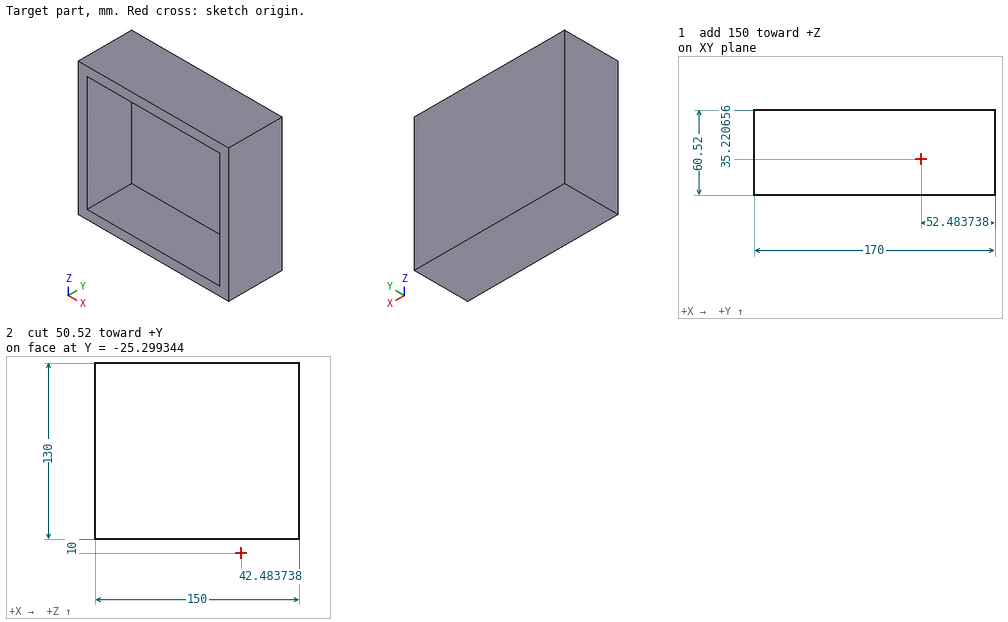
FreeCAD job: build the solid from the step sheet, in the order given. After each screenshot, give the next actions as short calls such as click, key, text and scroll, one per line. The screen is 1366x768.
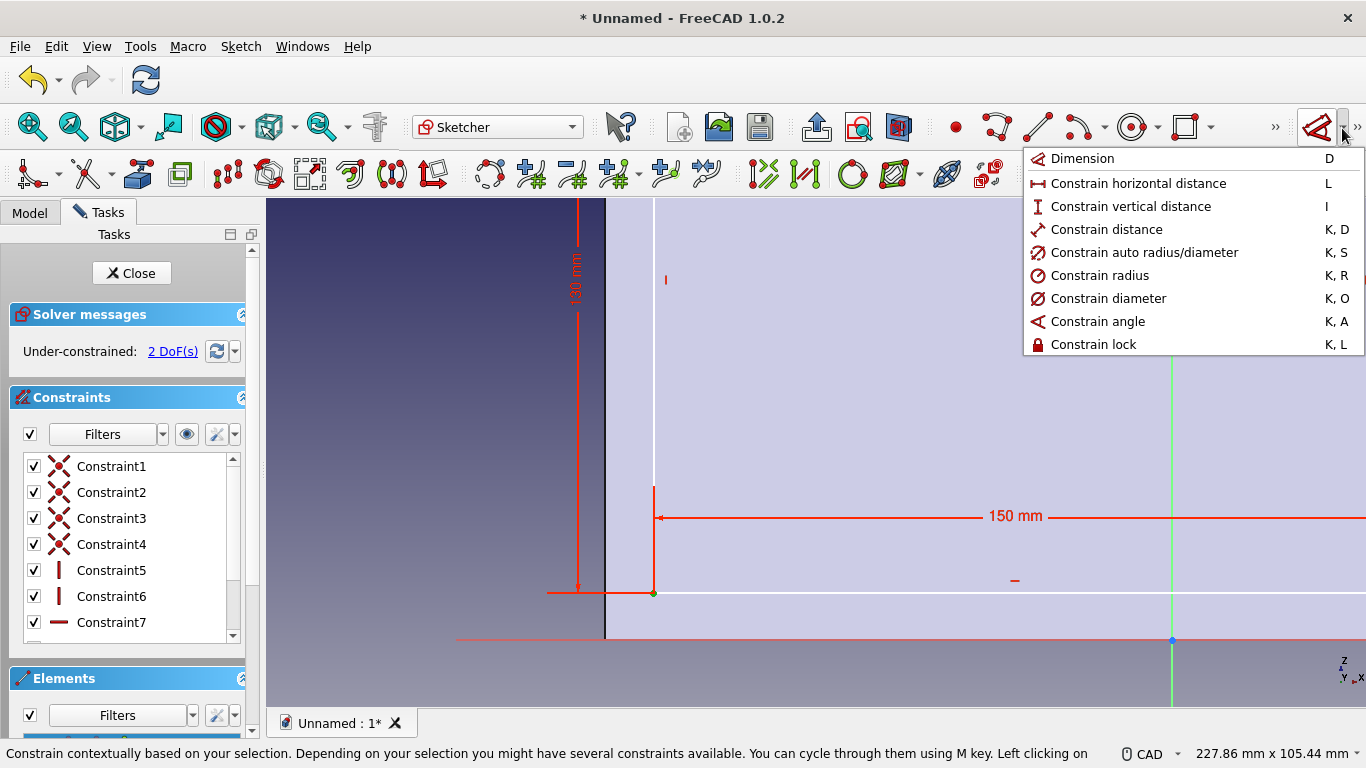
click(1194, 206)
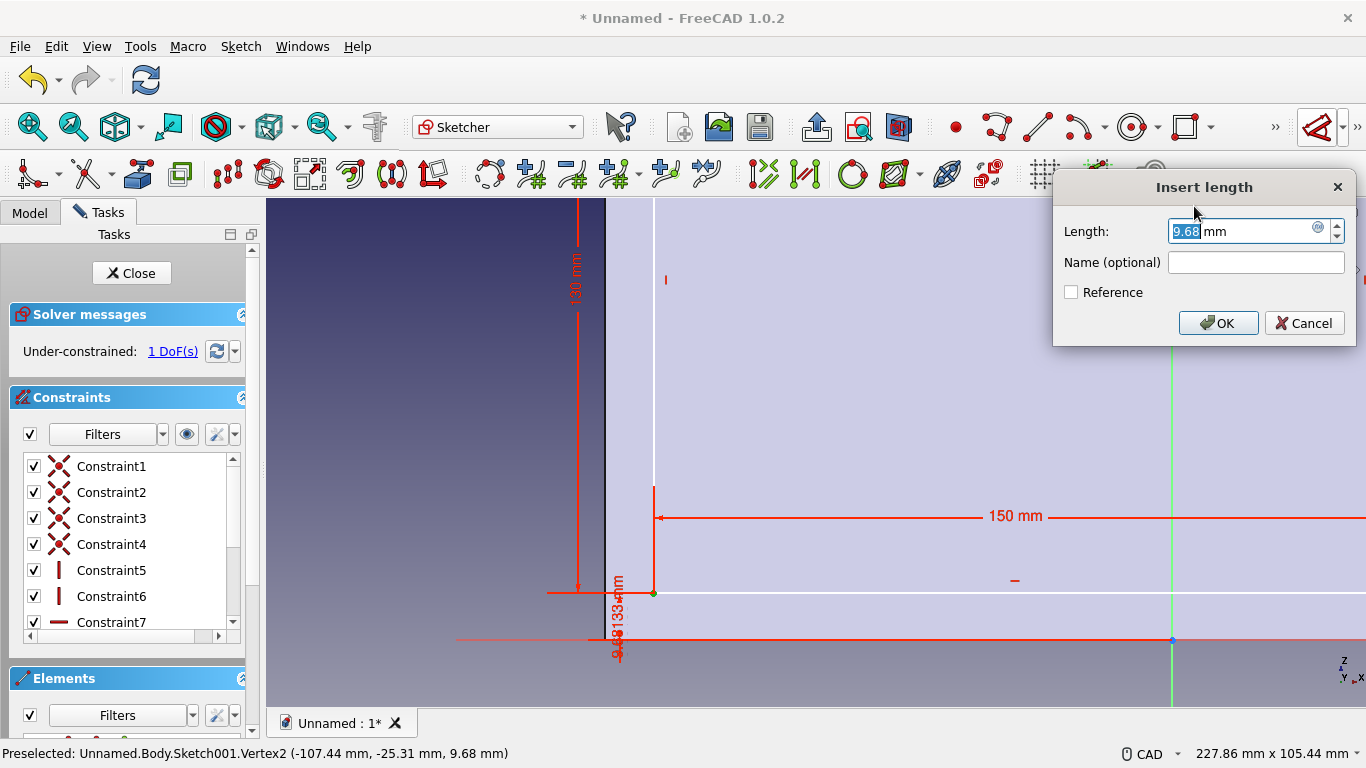
text(10)
key(Return)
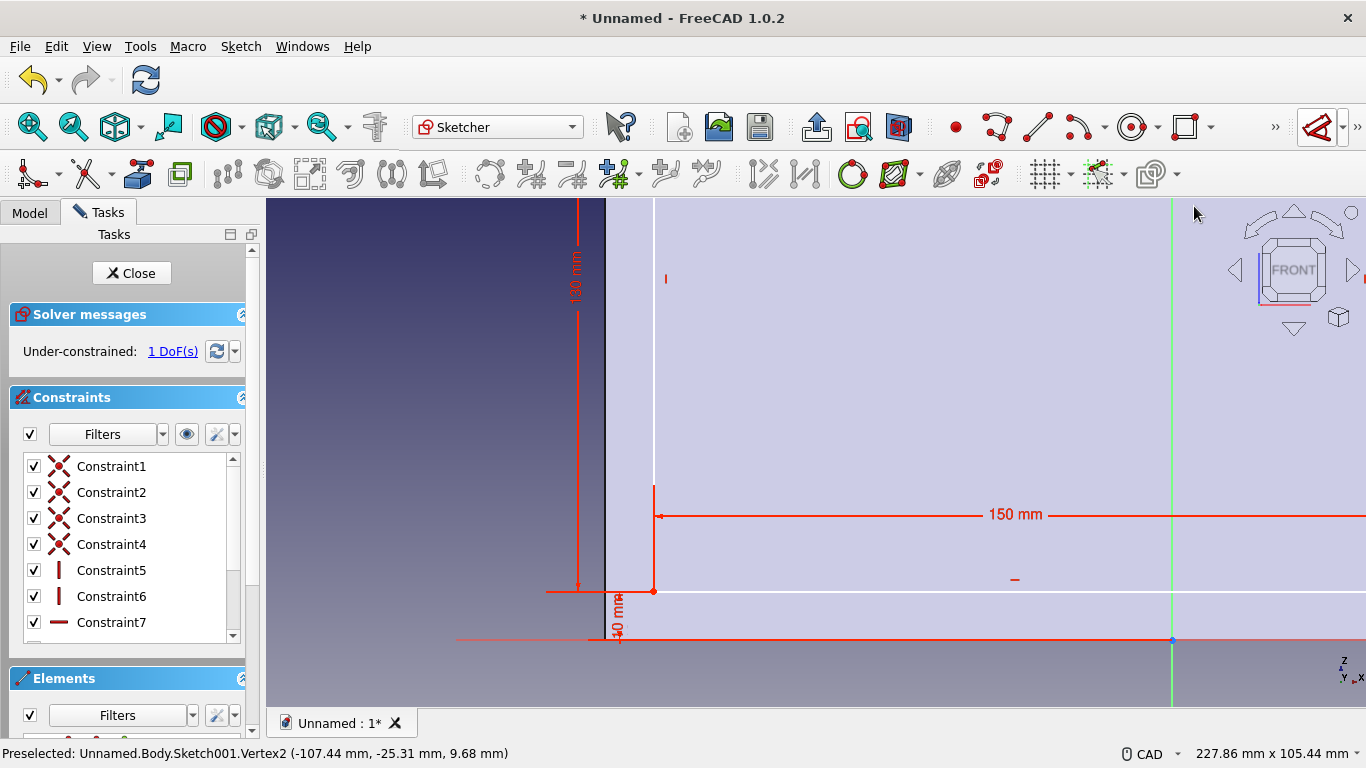
scroll(529, 575, down, 4)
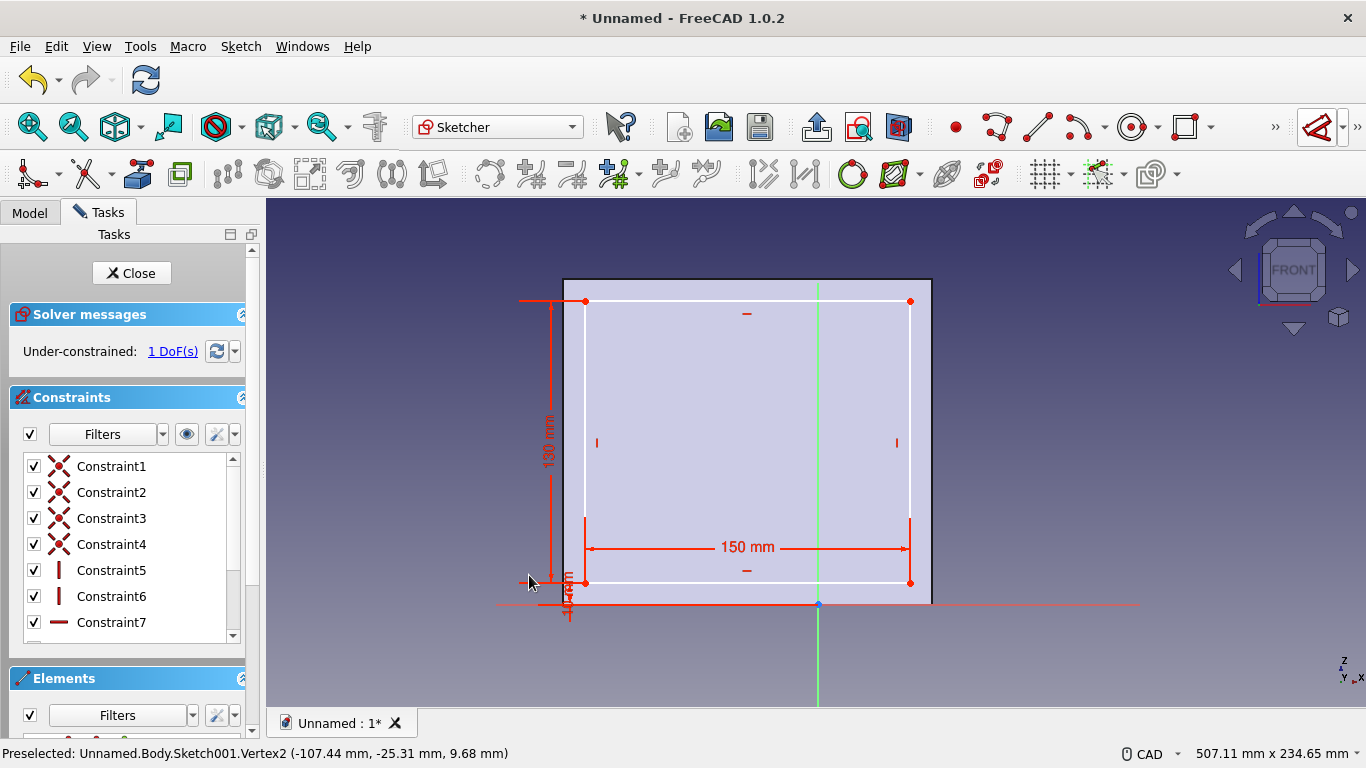
click(911, 583)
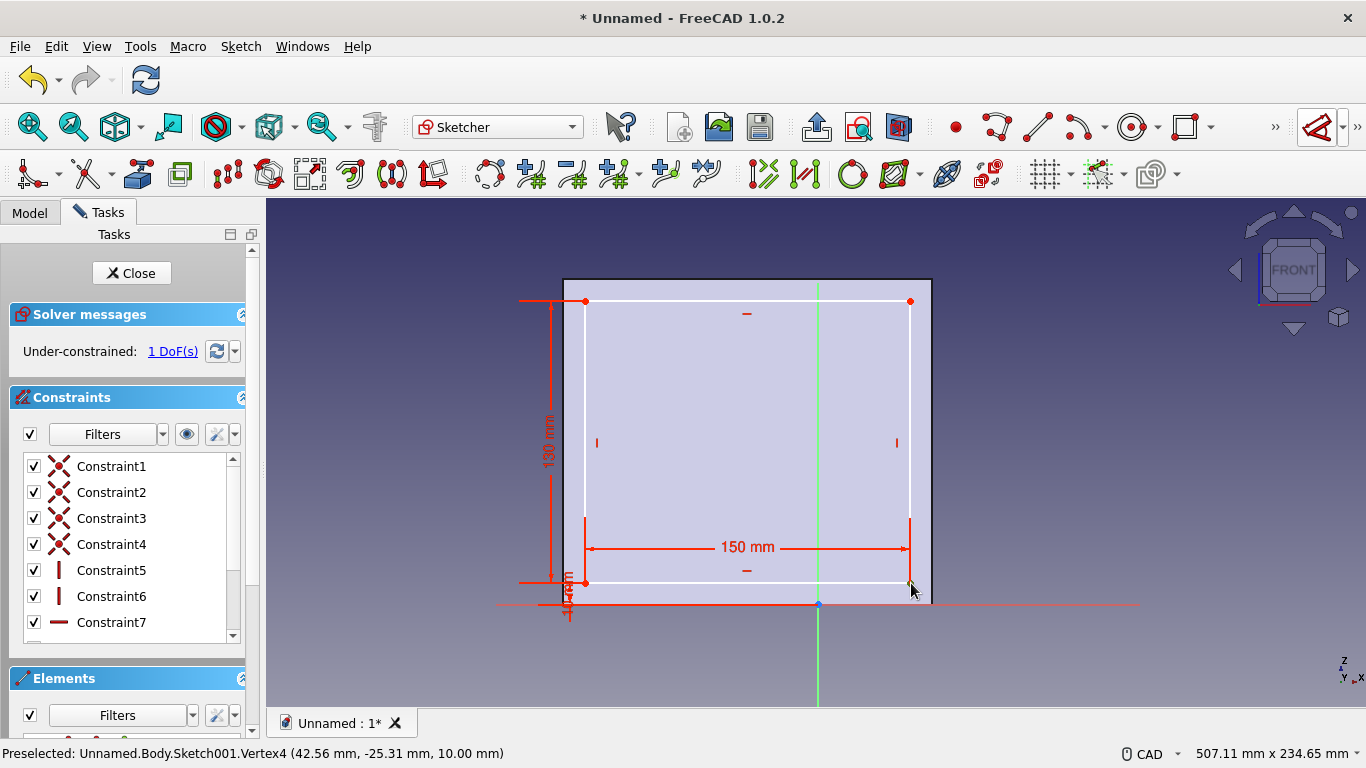
key(l)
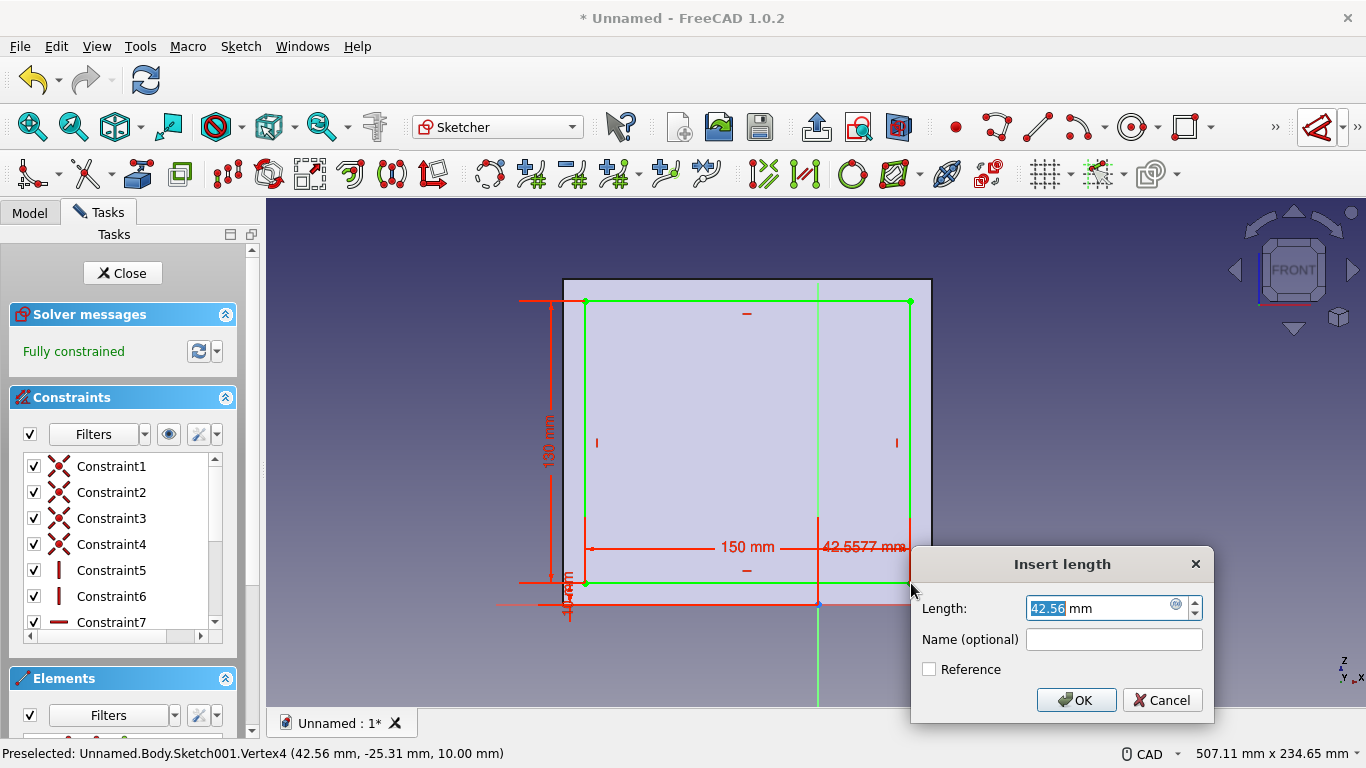
text(42.483738)
key(Return)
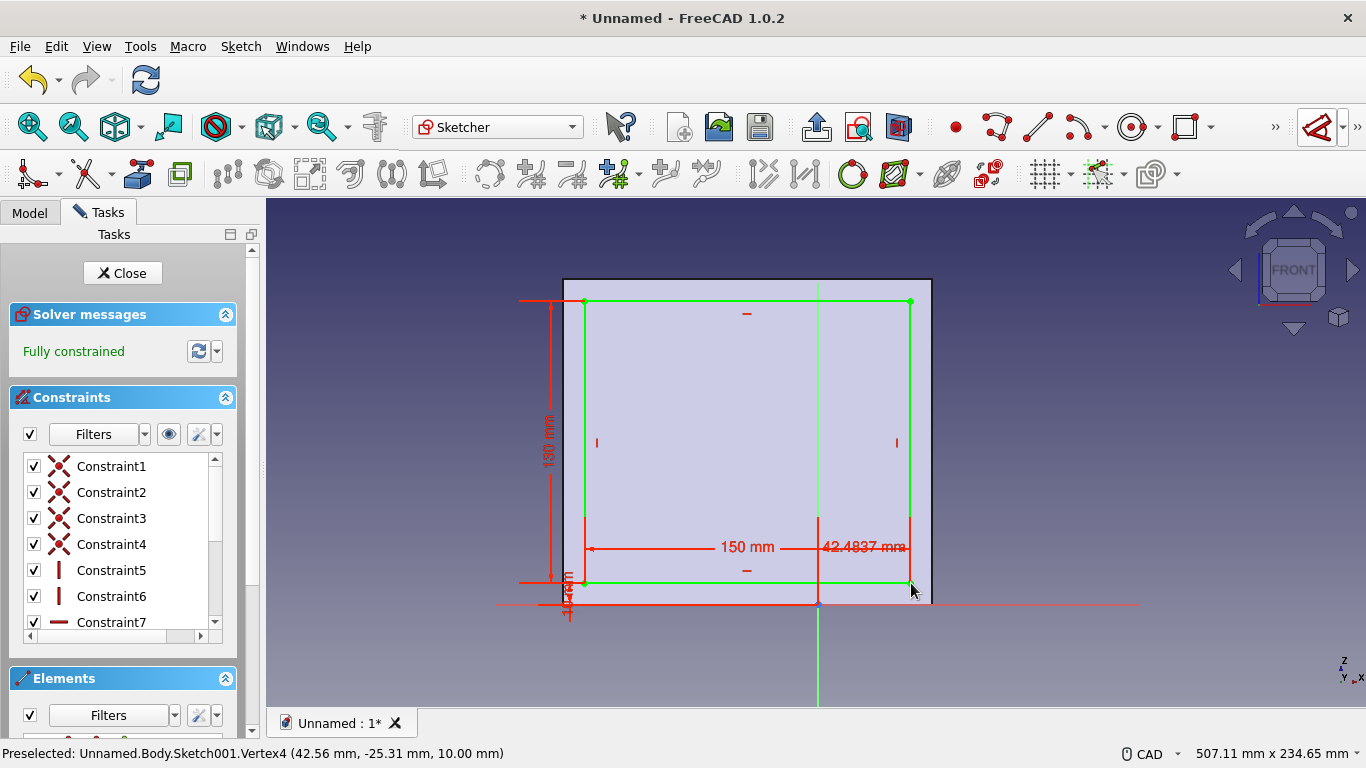
click(123, 273)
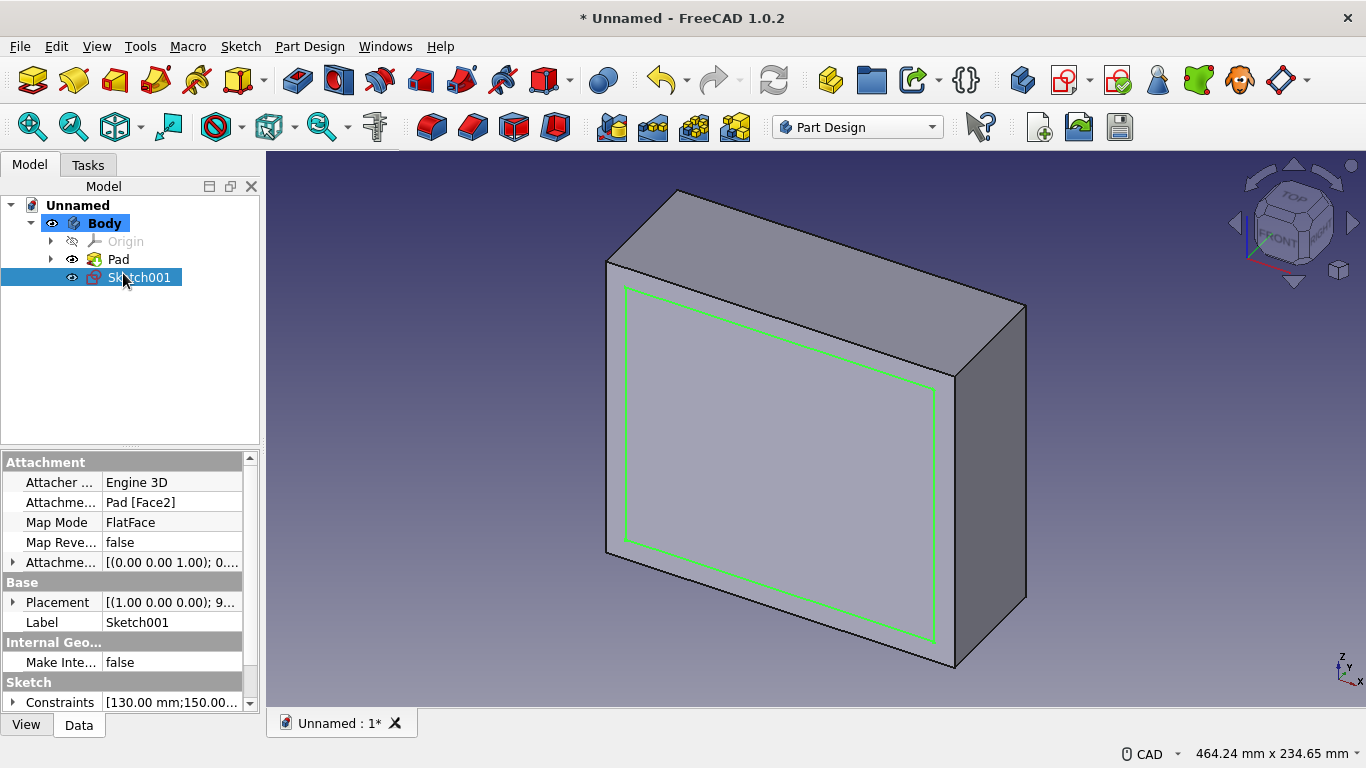
click(298, 80)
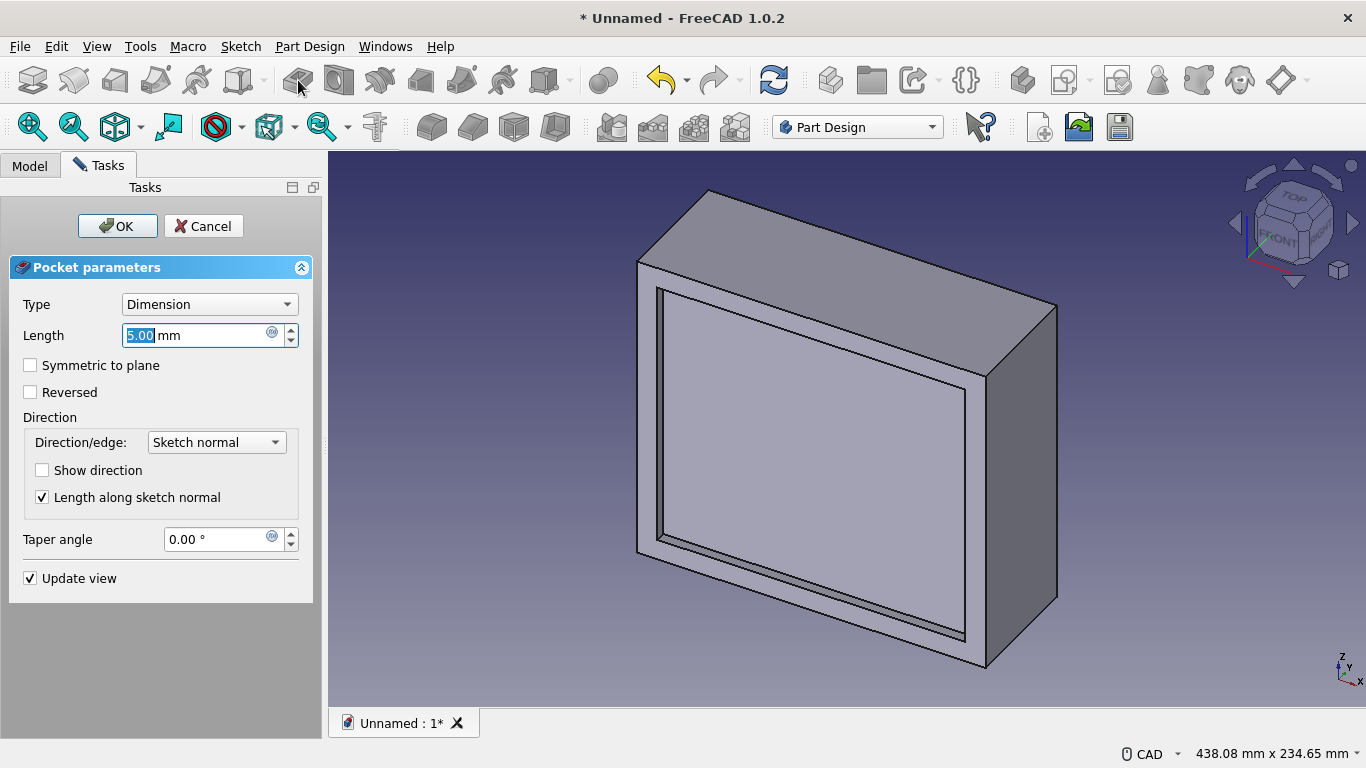
text(50.52)
key(Tab)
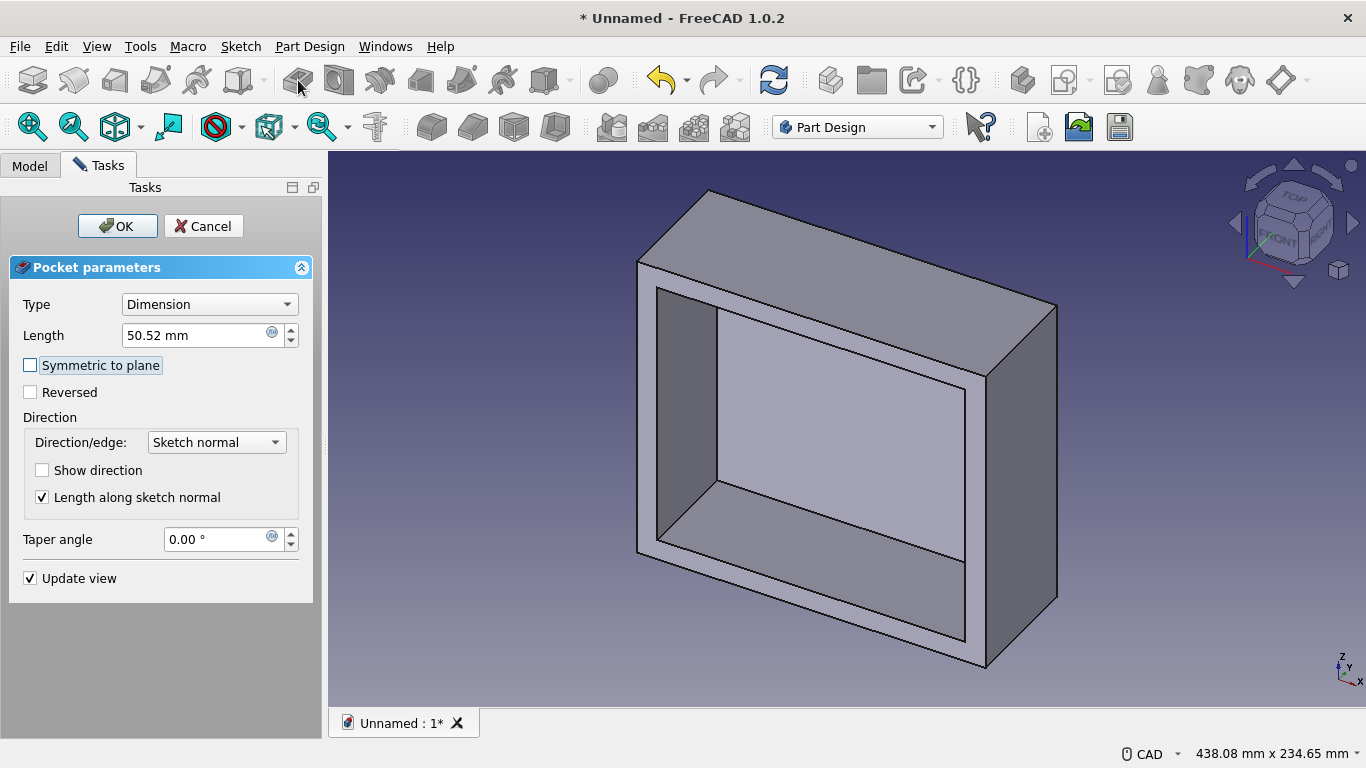
click(118, 226)